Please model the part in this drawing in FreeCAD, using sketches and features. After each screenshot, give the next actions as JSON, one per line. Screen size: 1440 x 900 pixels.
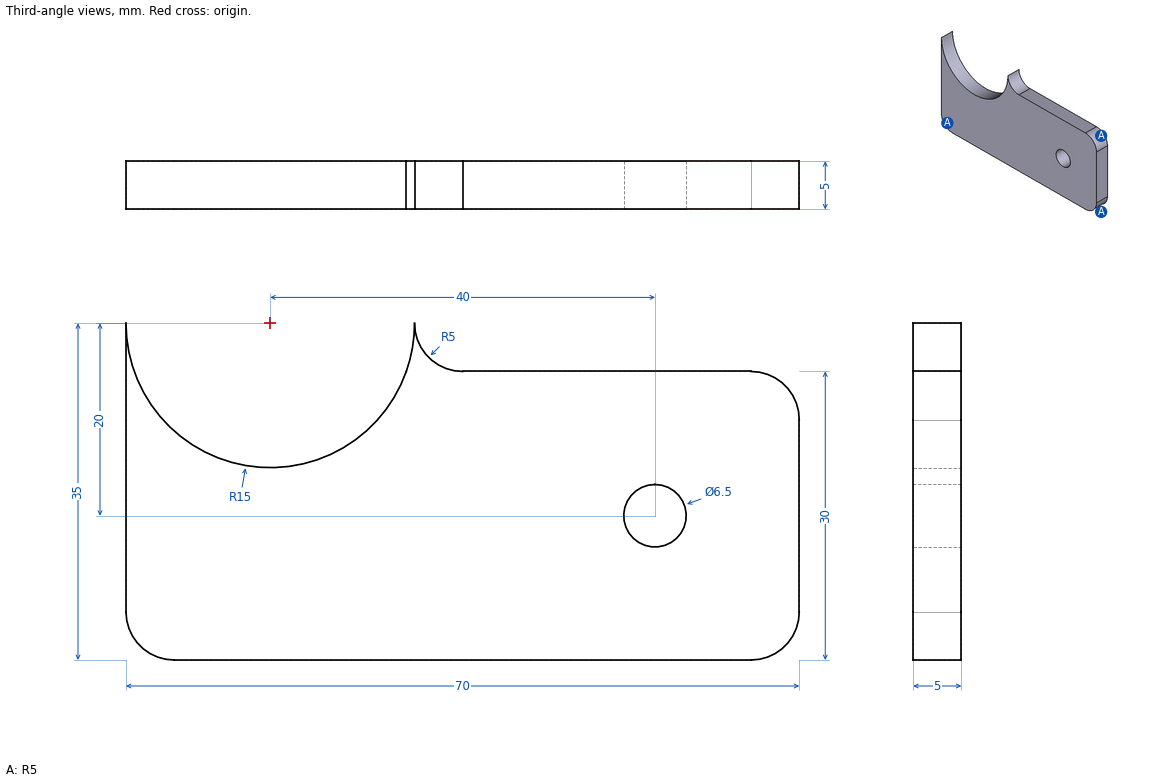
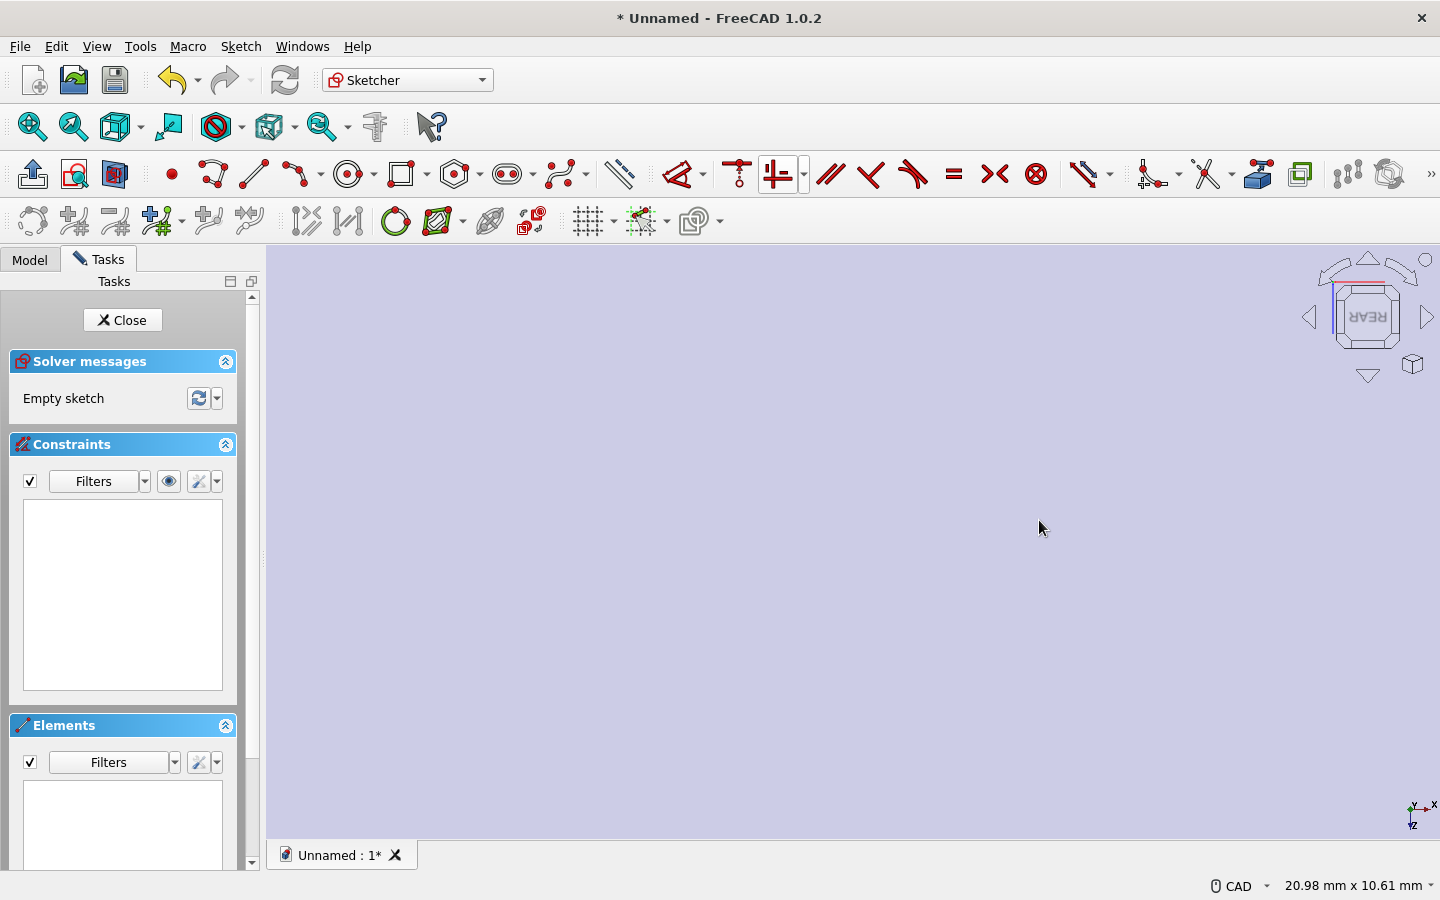
{"action": "left_click", "coordinate": [348, 174]}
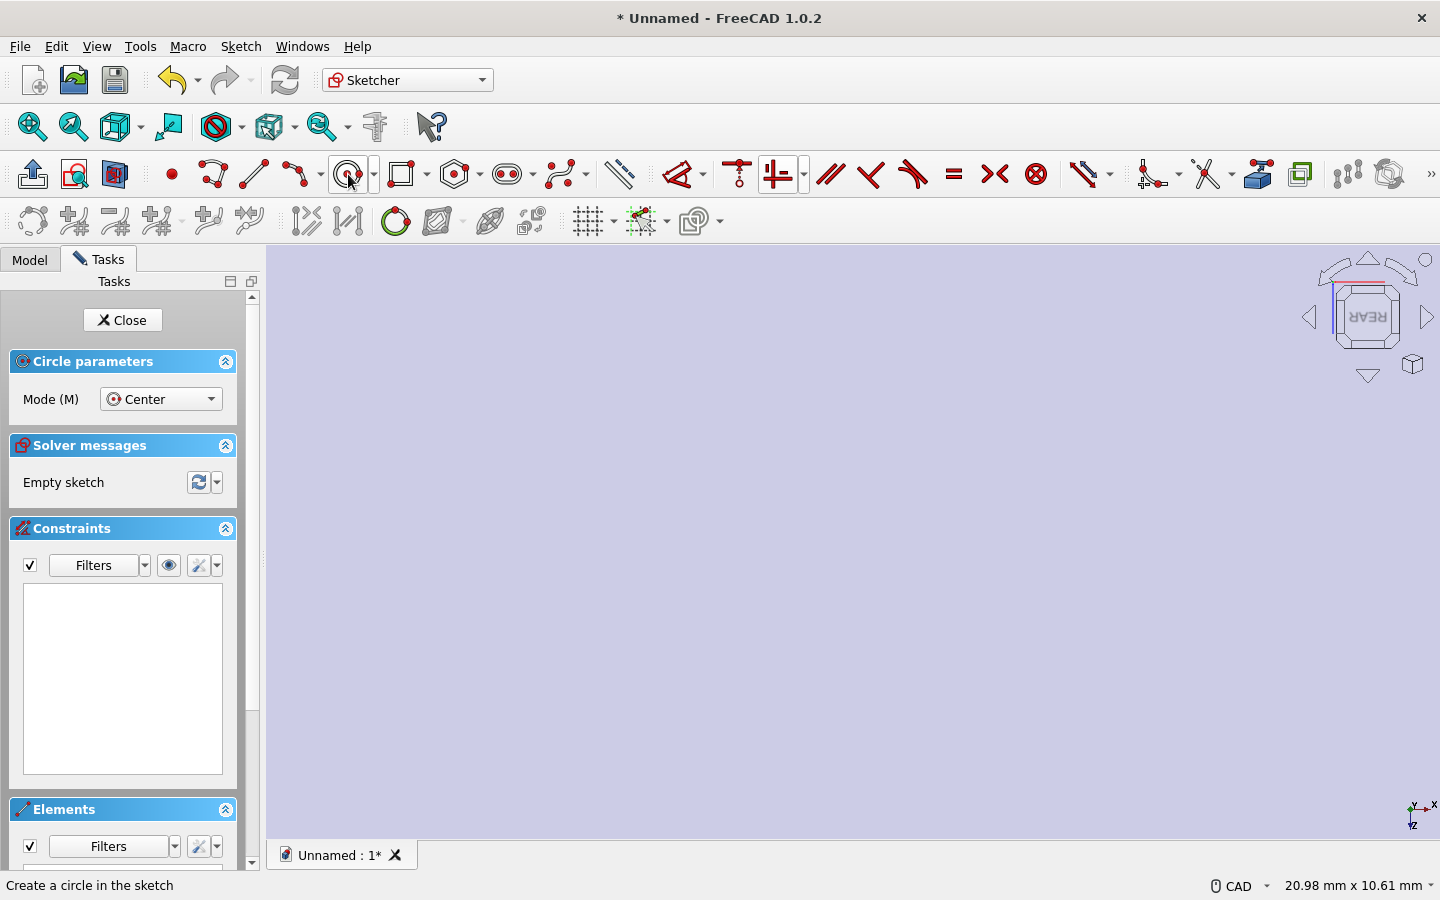
{"action": "left_click", "coordinate": [780, 540]}
{"action": "mouse_move", "coordinate": [908, 411]}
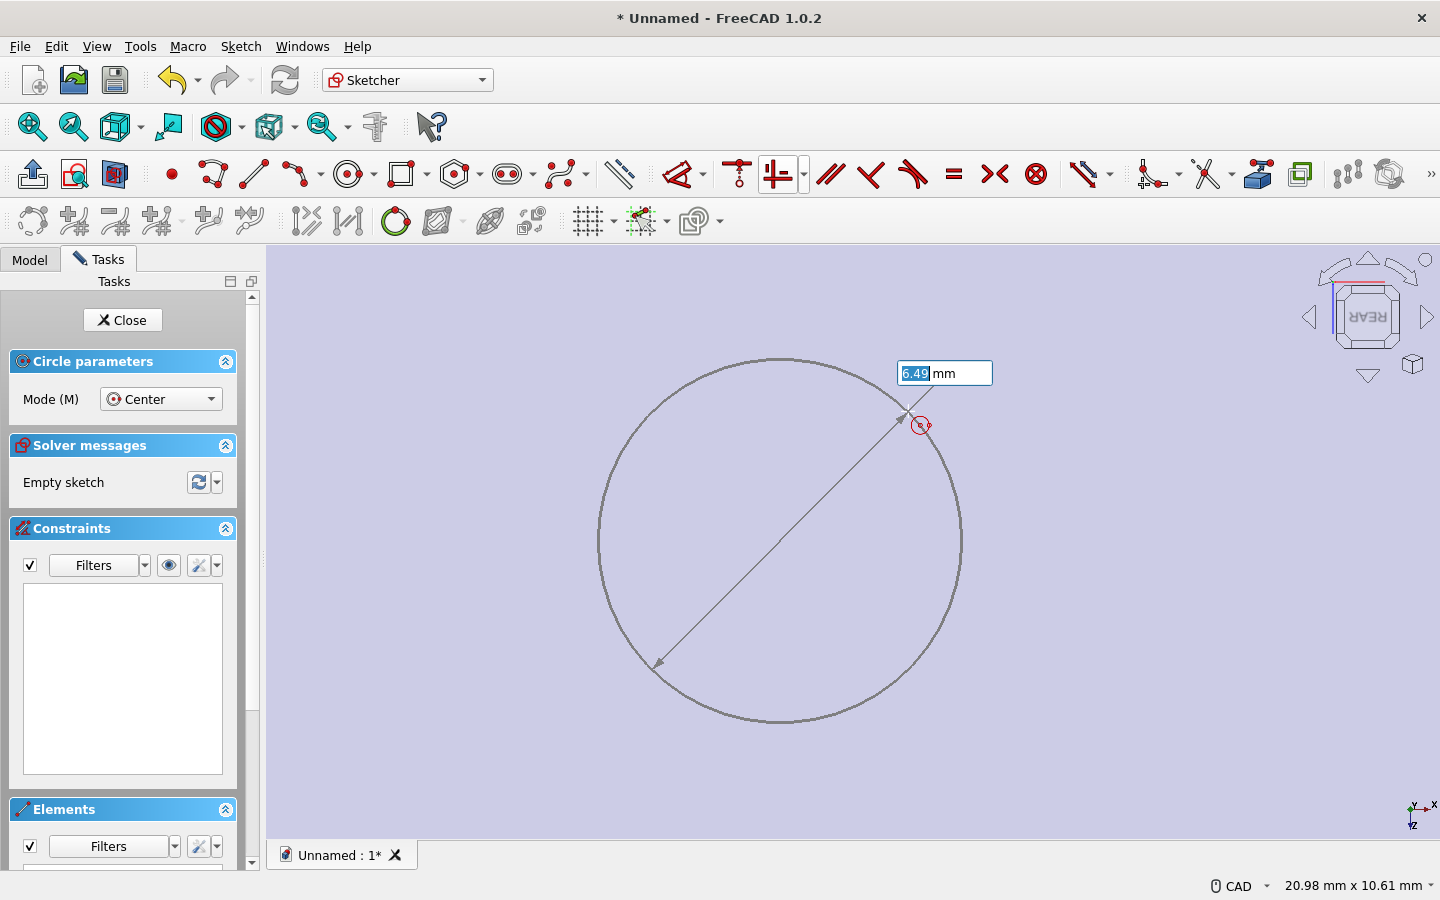
{"action": "type", "text": "6.5"}
{"action": "key", "text": "Return"}
{"action": "key", "text": "Escape"}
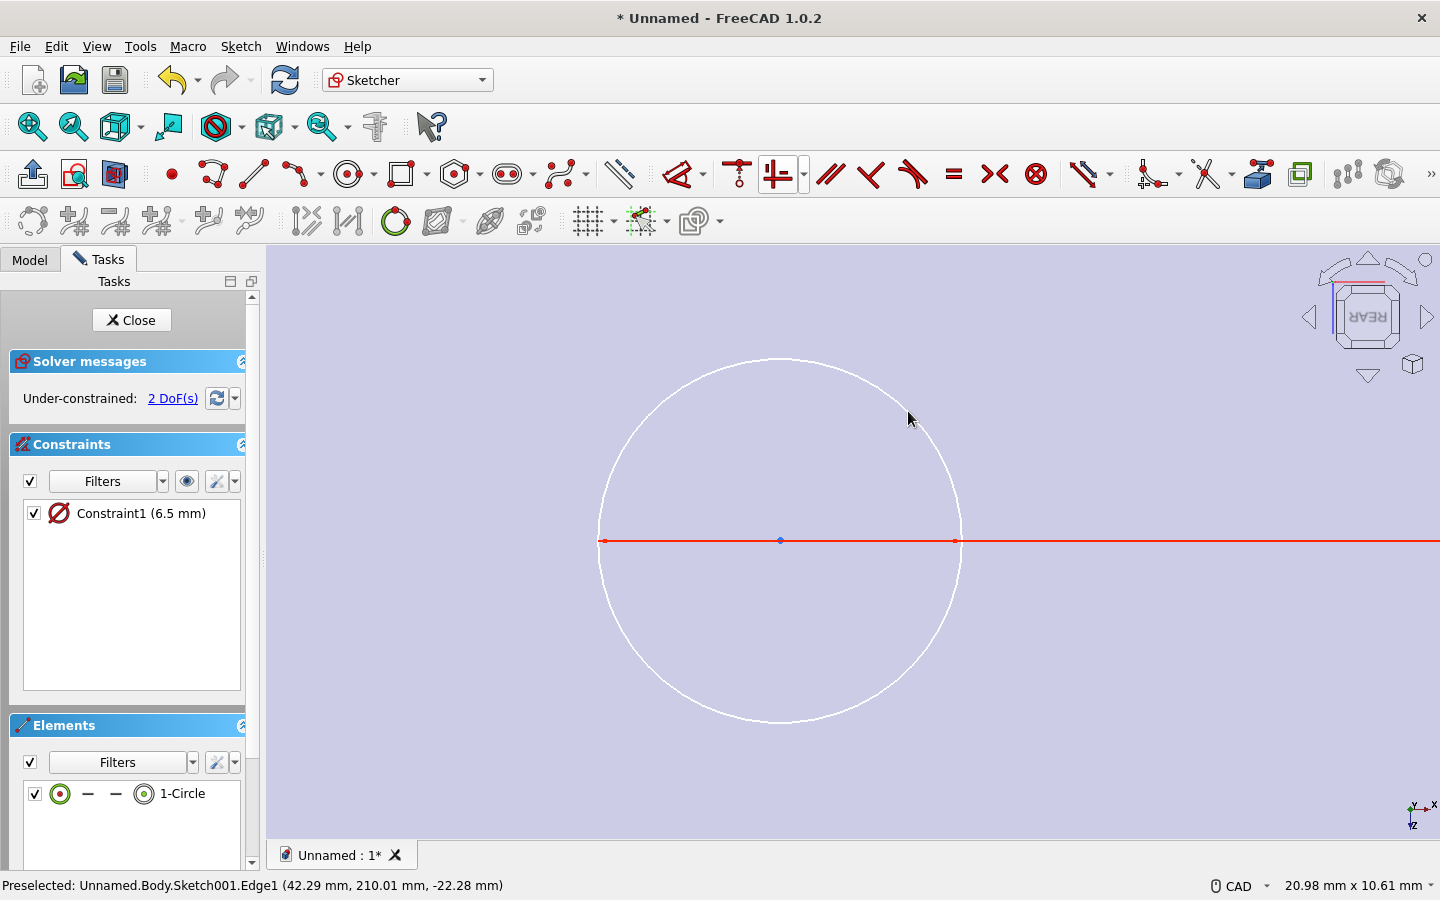
{"action": "left_click", "coordinate": [676, 174]}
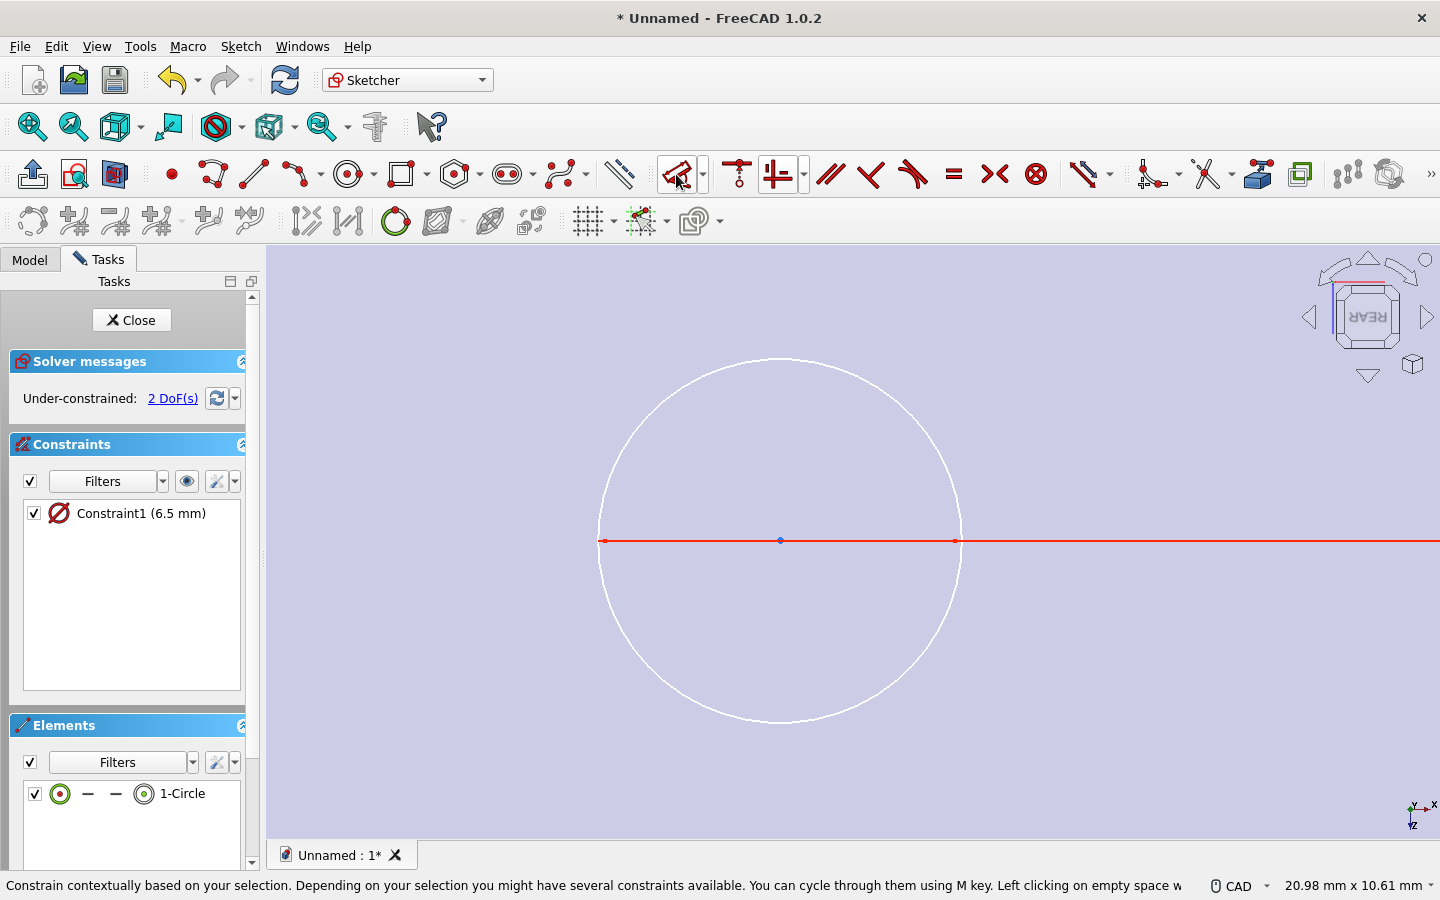
{"action": "left_click", "coordinate": [780, 541]}
{"action": "left_click", "coordinate": [537, 507]}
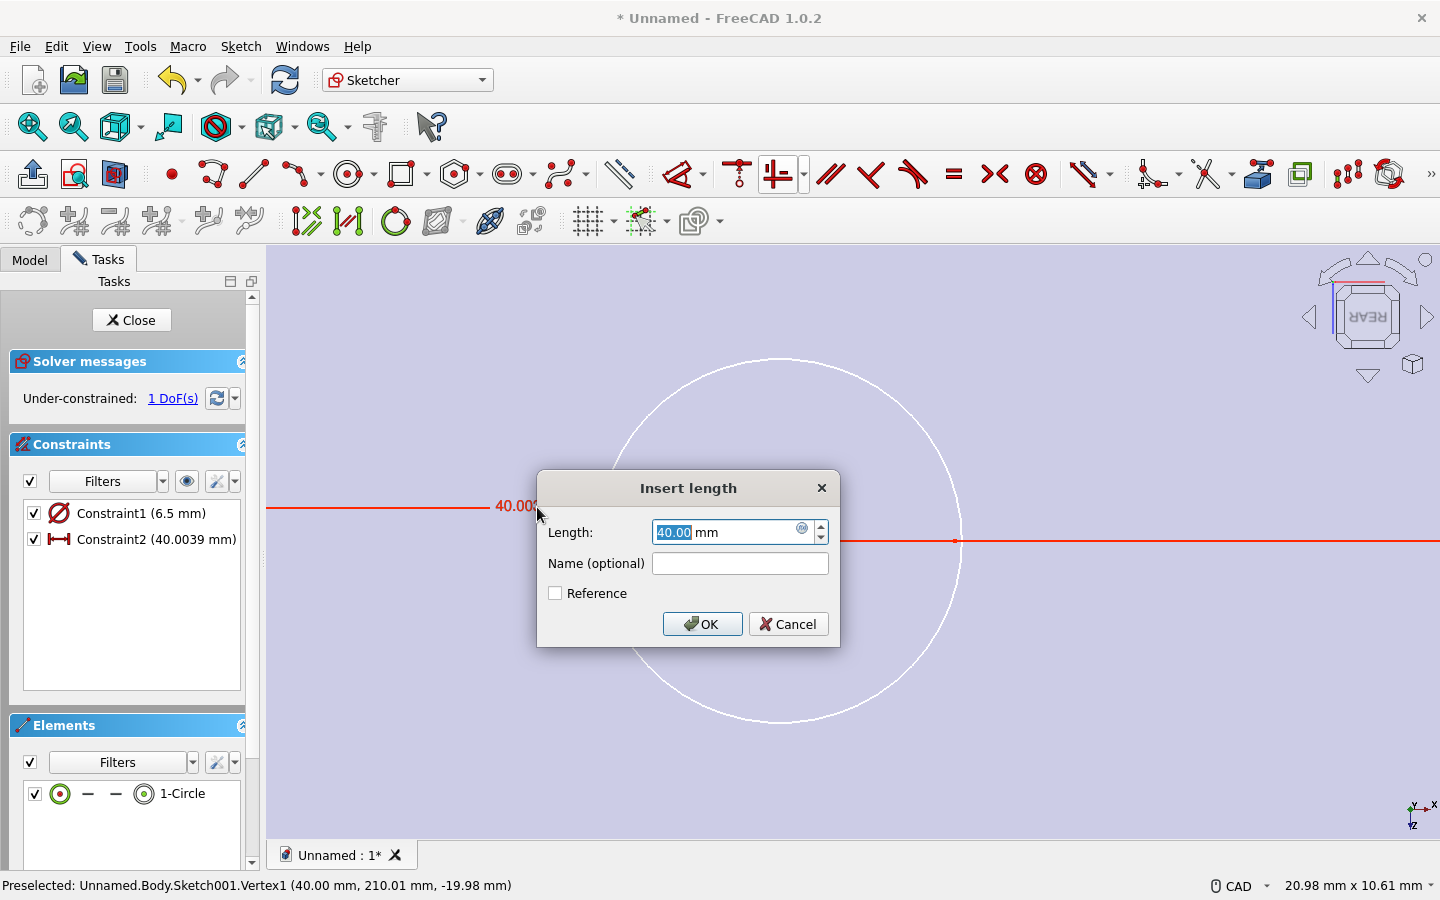
{"action": "type", "text": "40"}
{"action": "key", "text": "Return"}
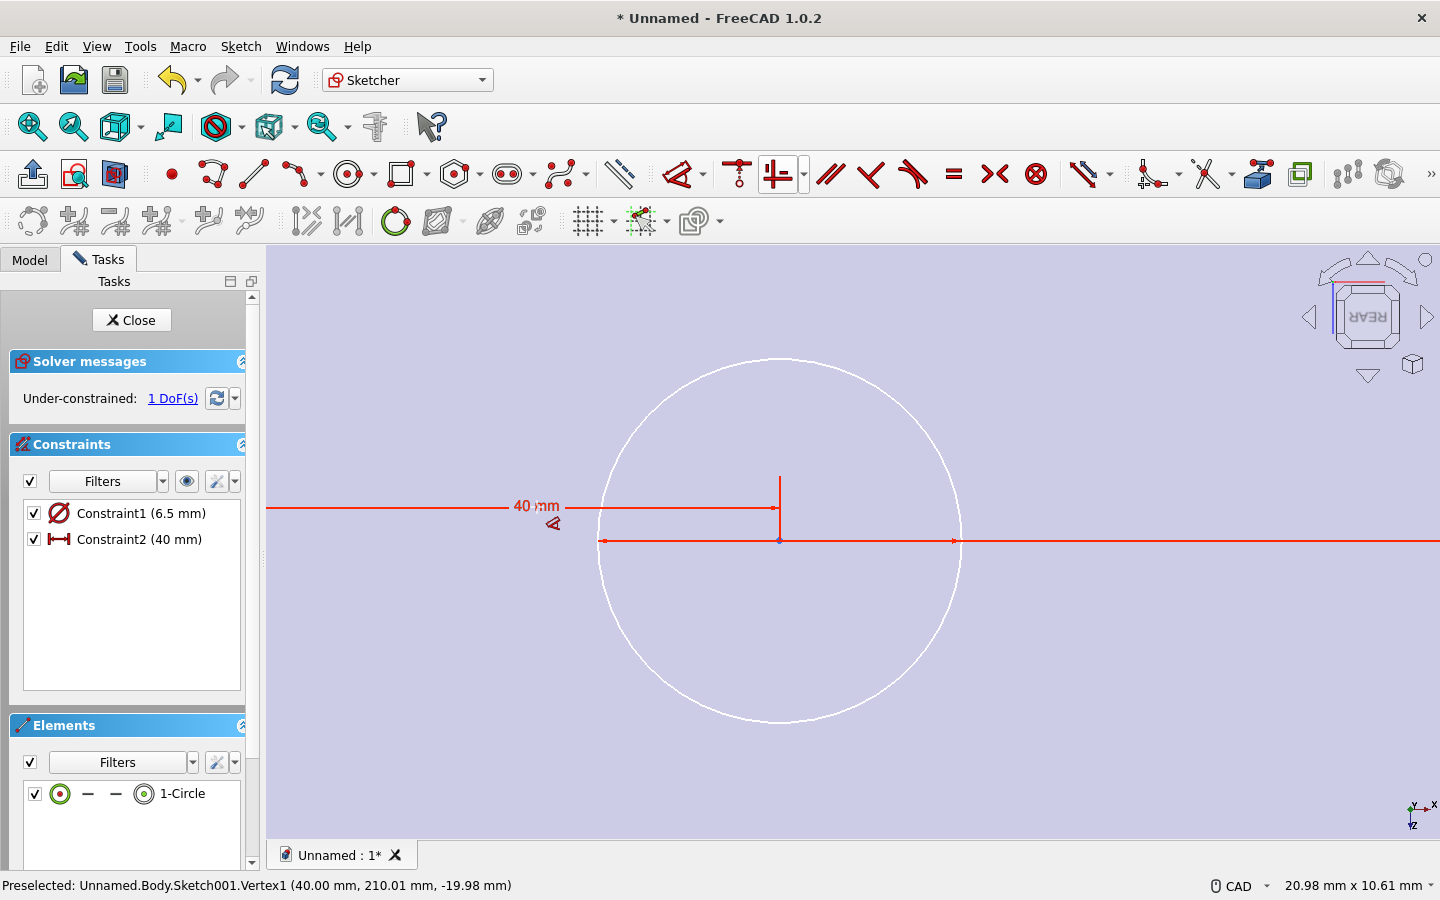
{"action": "left_click", "coordinate": [780, 541]}
{"action": "left_click", "coordinate": [814, 676]}